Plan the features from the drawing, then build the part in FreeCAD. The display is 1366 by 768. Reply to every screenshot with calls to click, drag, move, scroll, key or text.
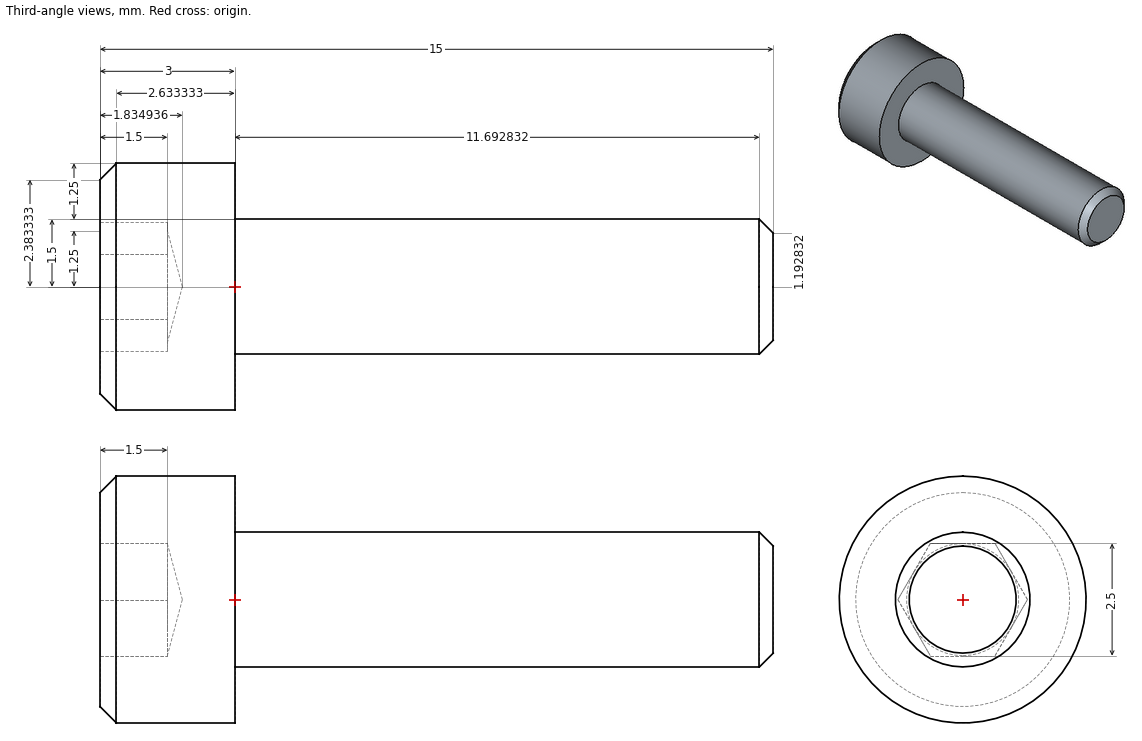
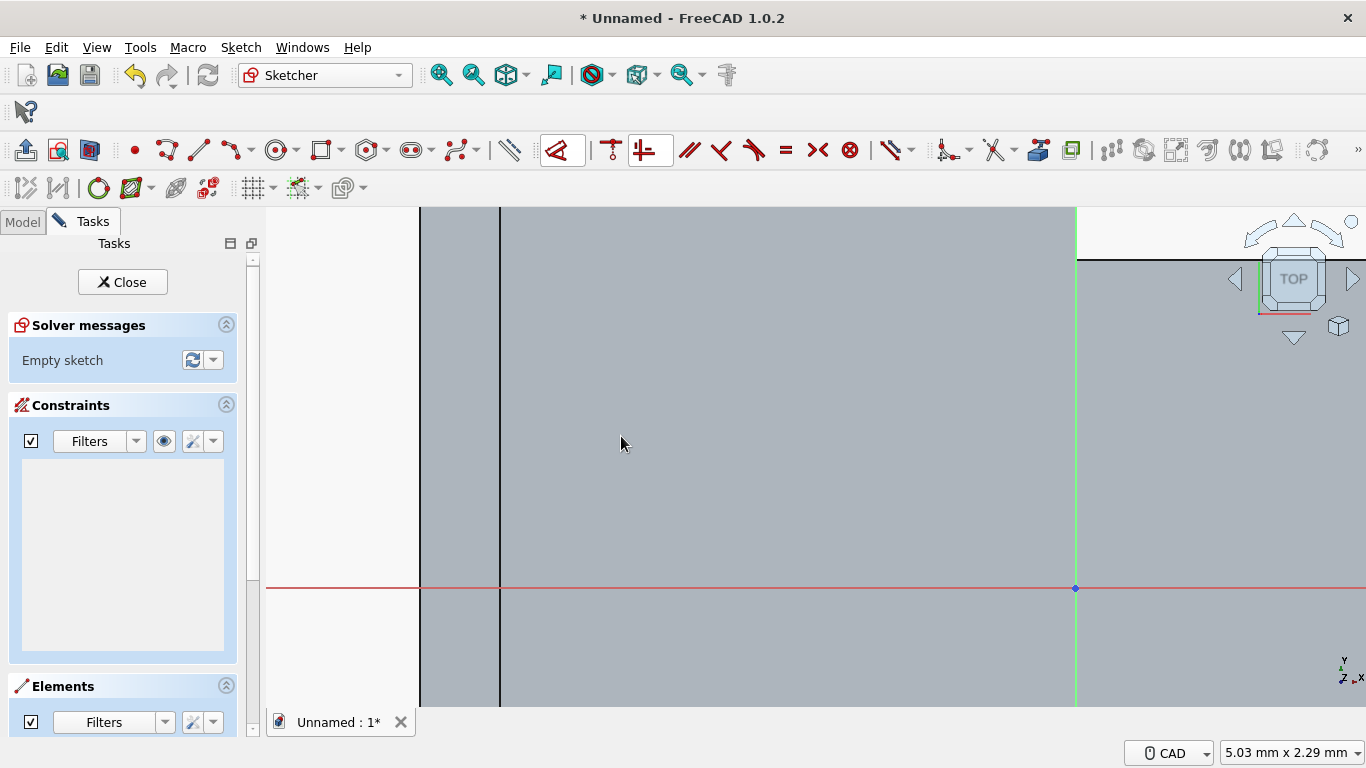
click(168, 150)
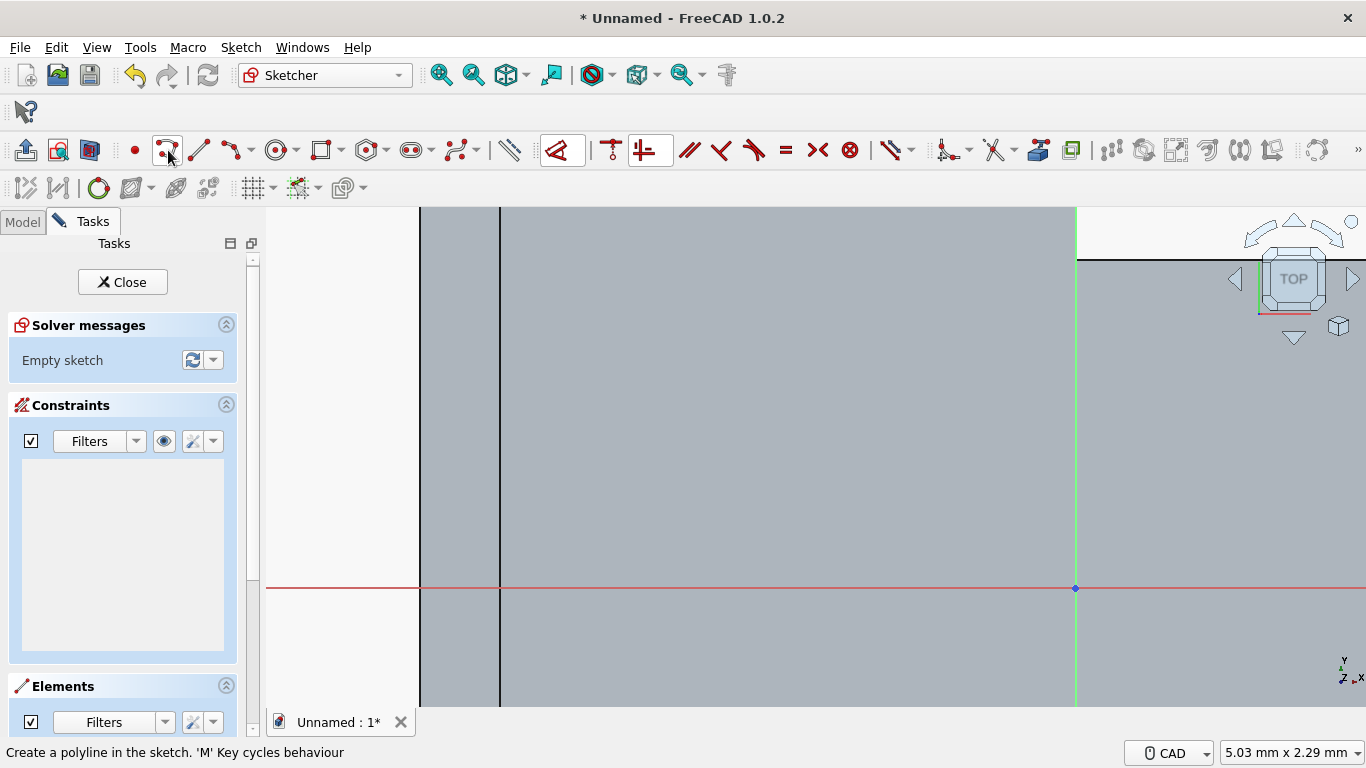
click(821, 588)
click(748, 315)
click(420, 315)
click(420, 579)
click(821, 588)
key(Escape)
key(Escape)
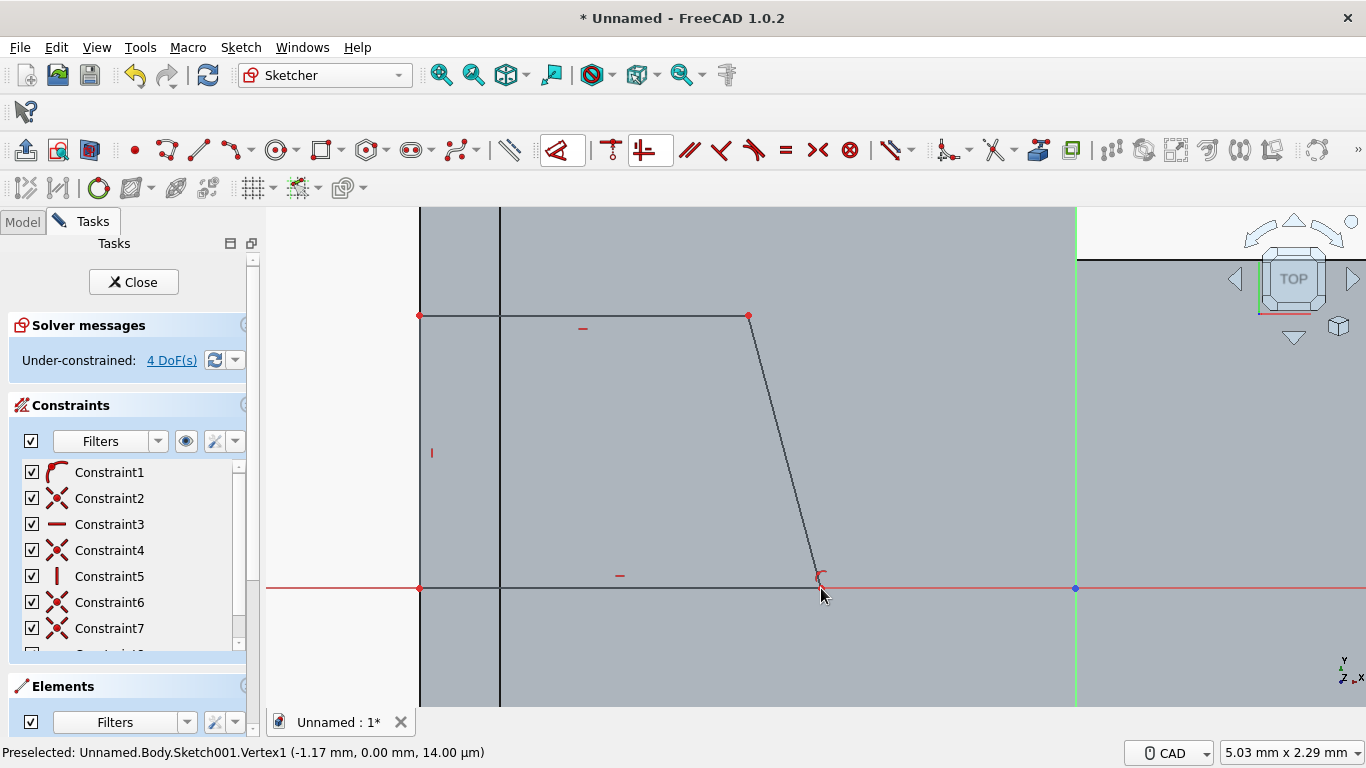
click(420, 316)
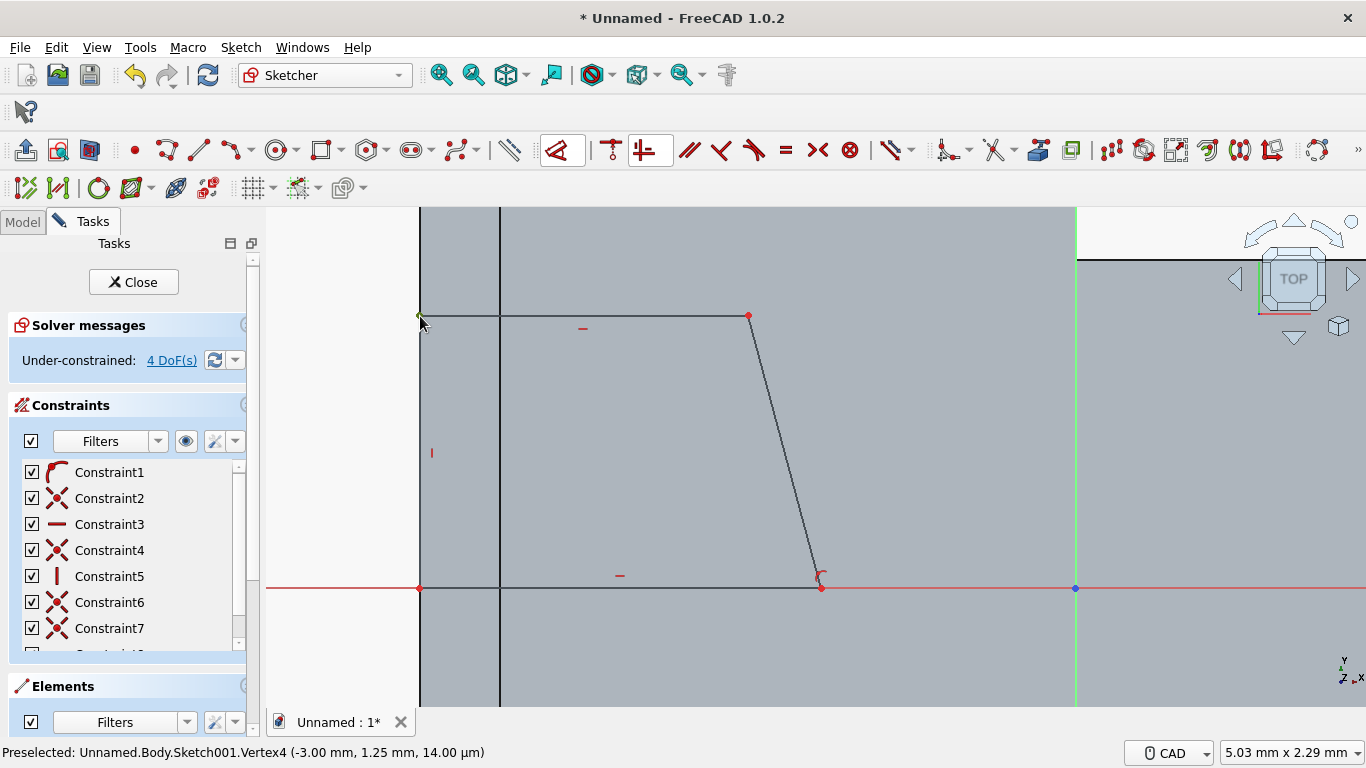
key(l)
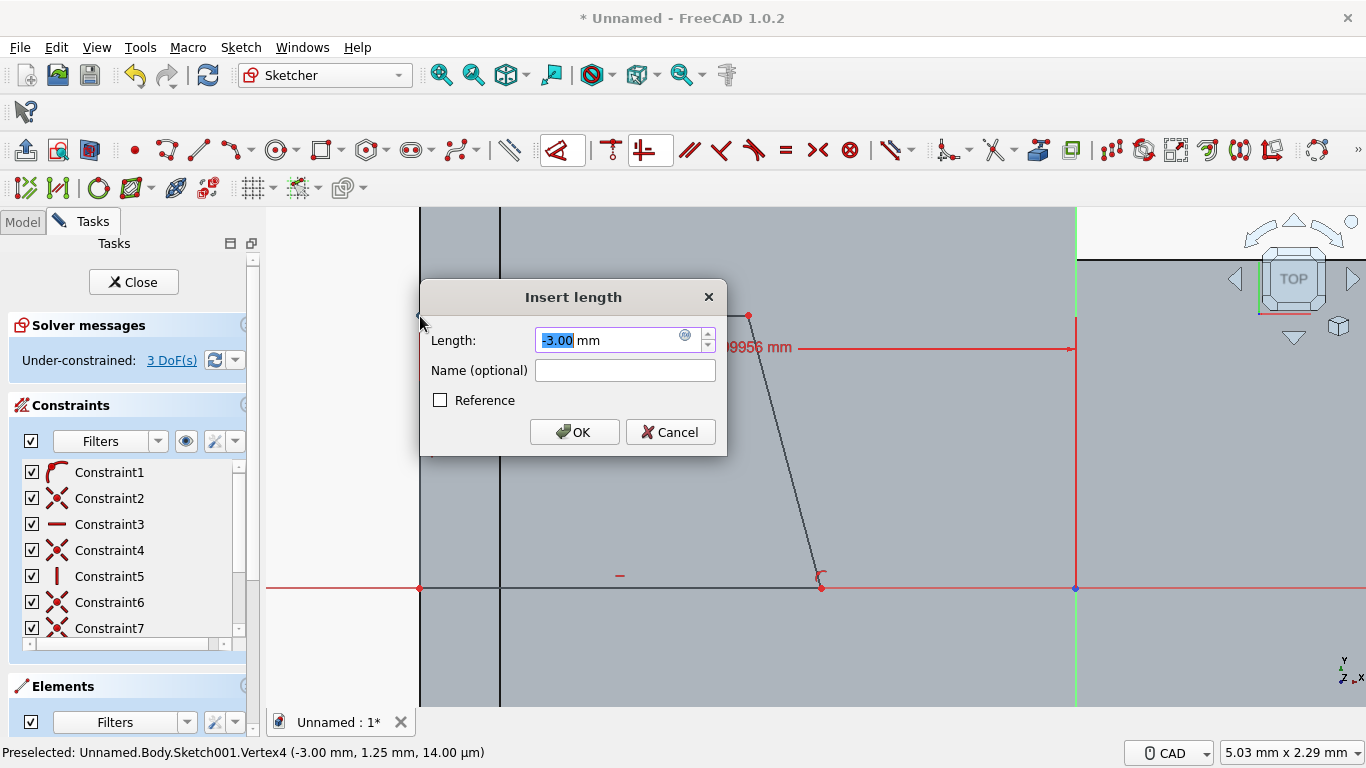
text(-3)
key(Return)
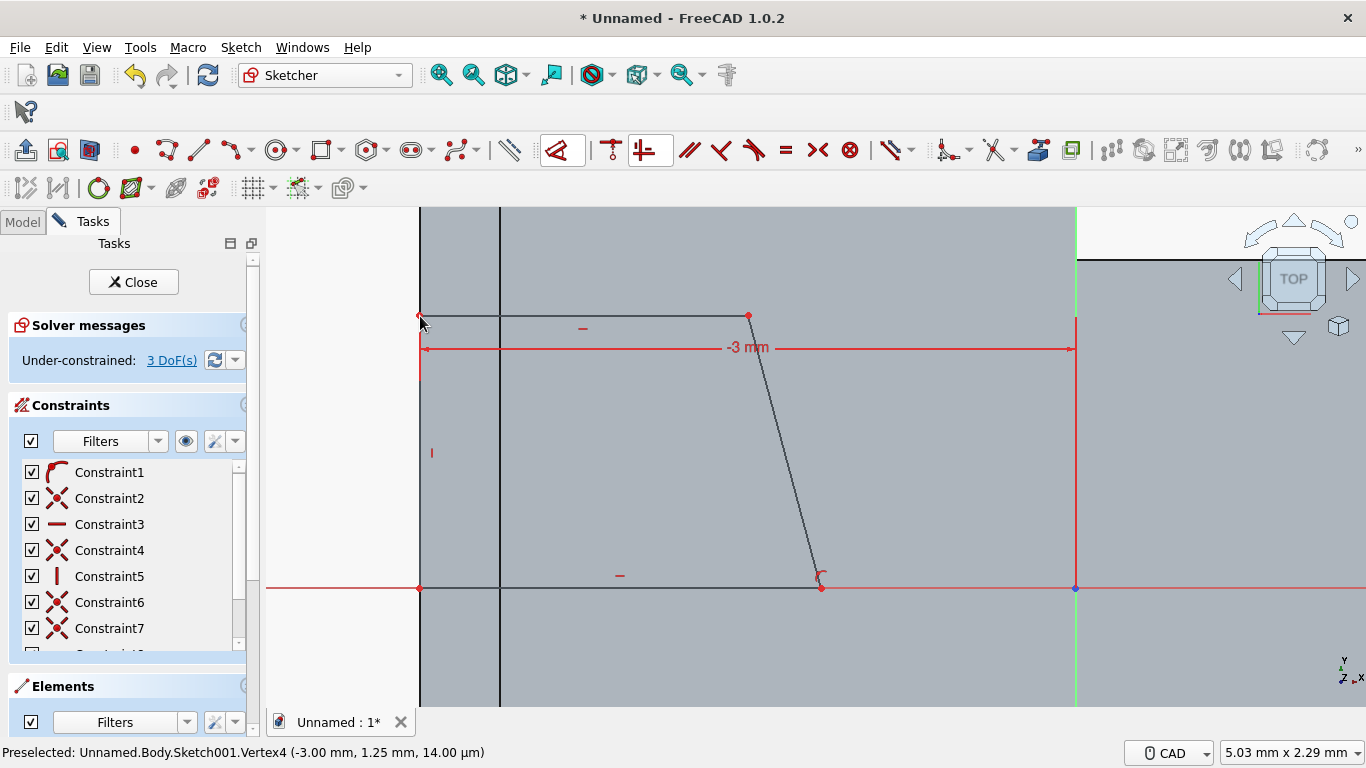
click(650, 316)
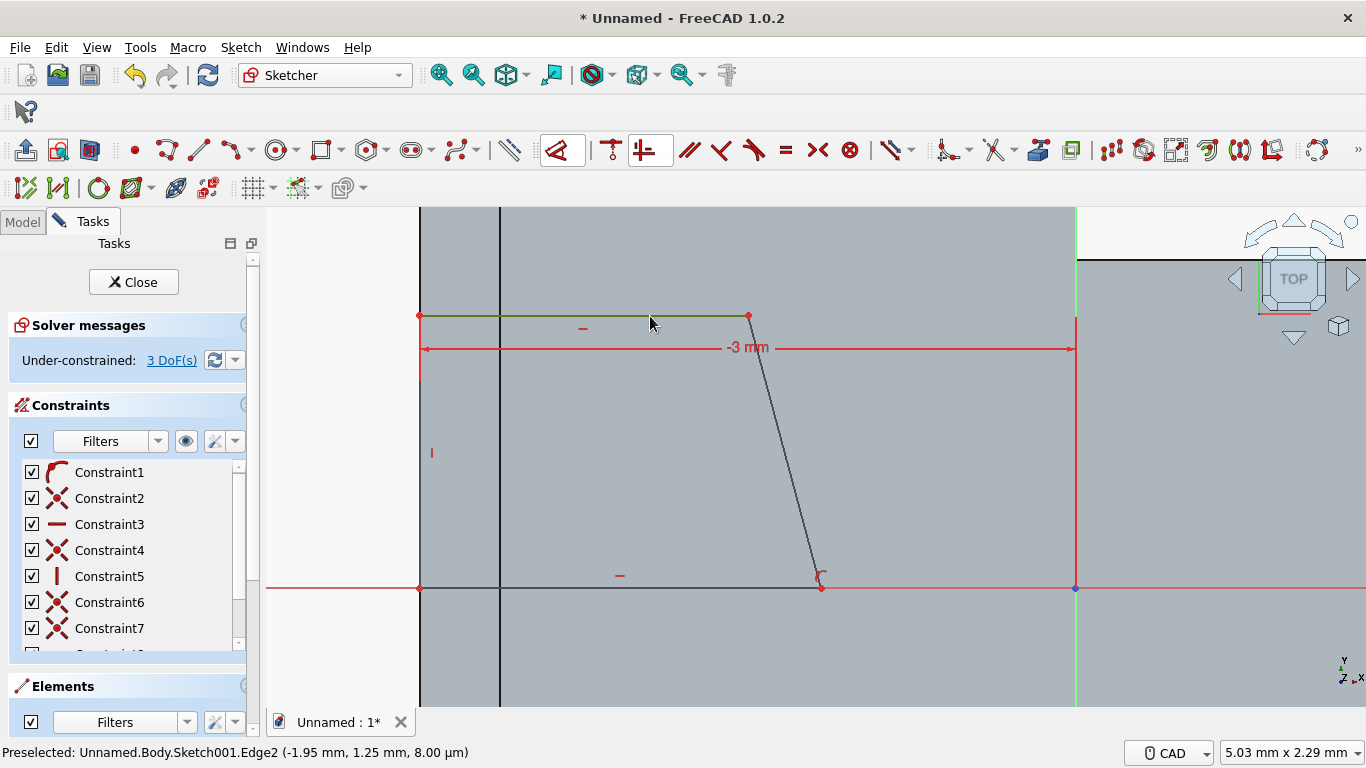
click(580, 150)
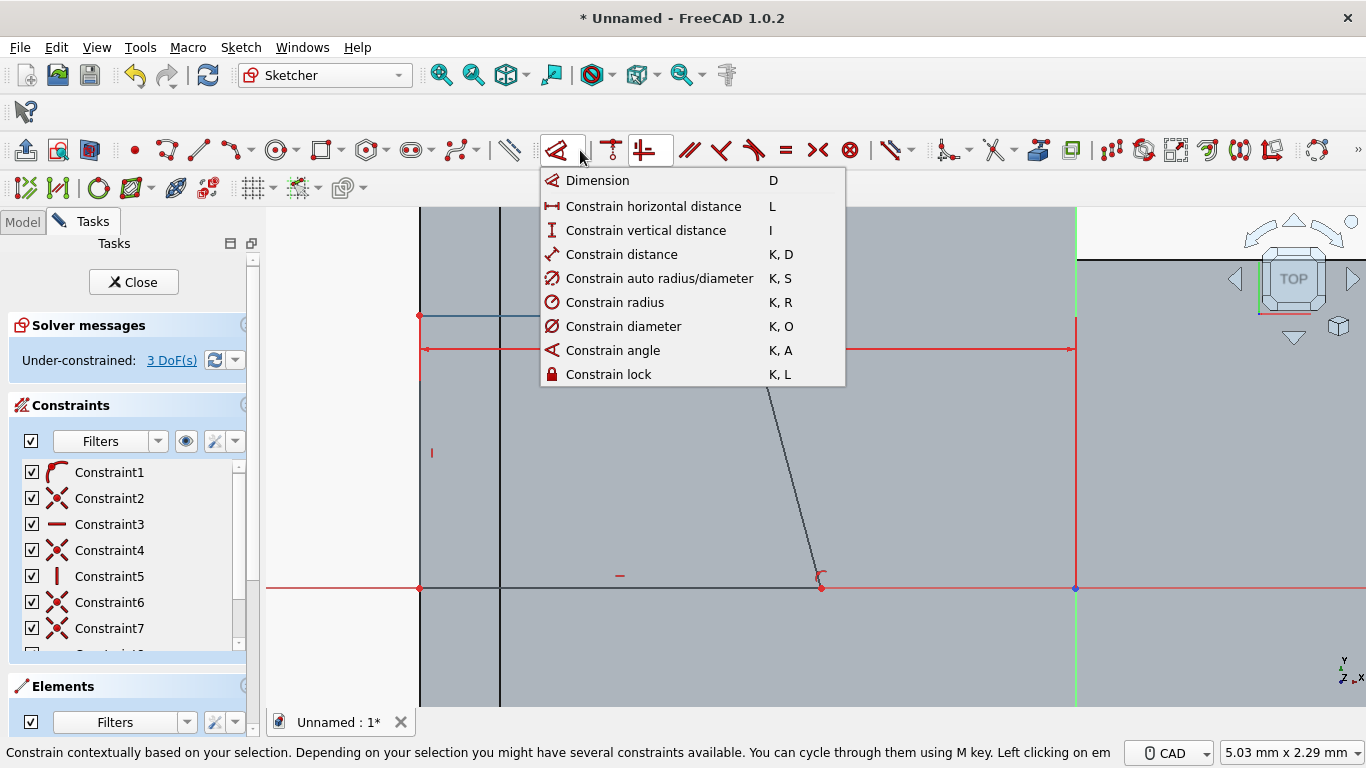
click(693, 206)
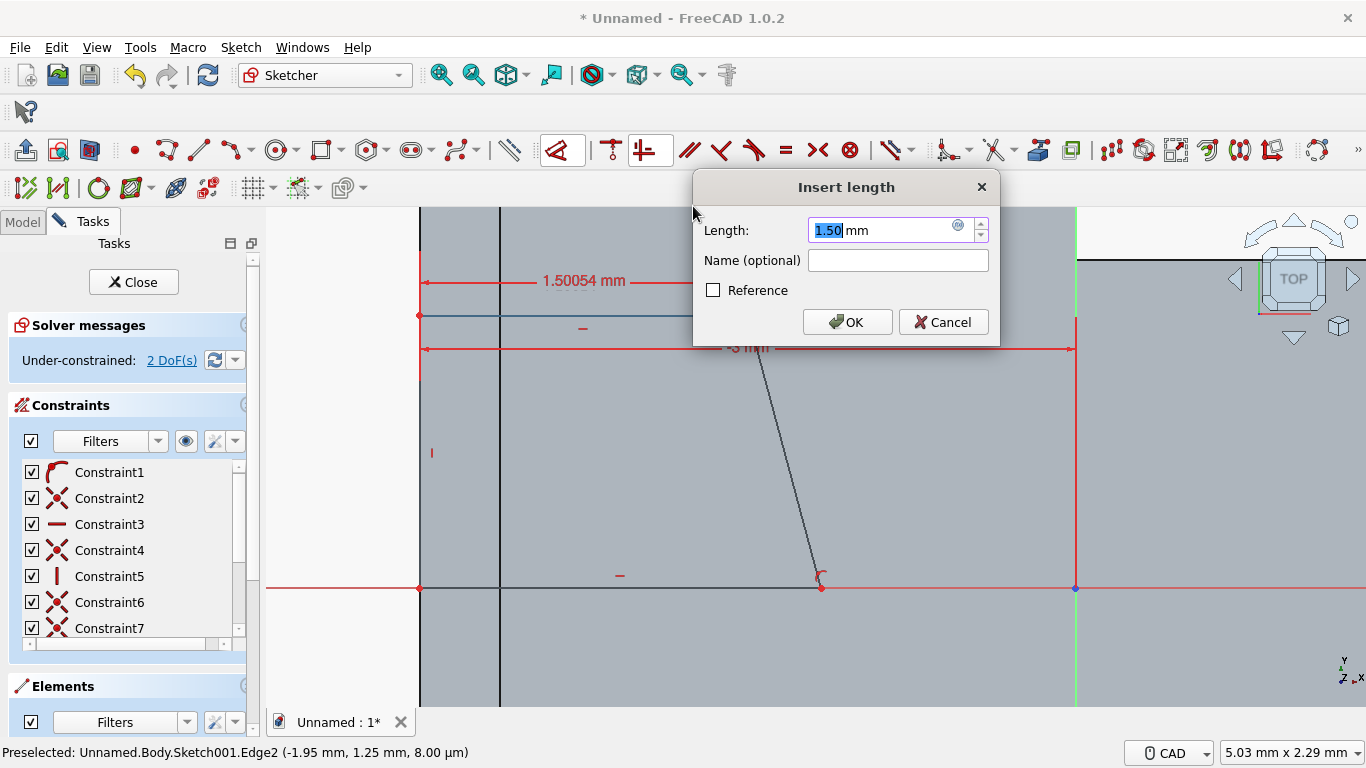
text(1.5)
key(Return)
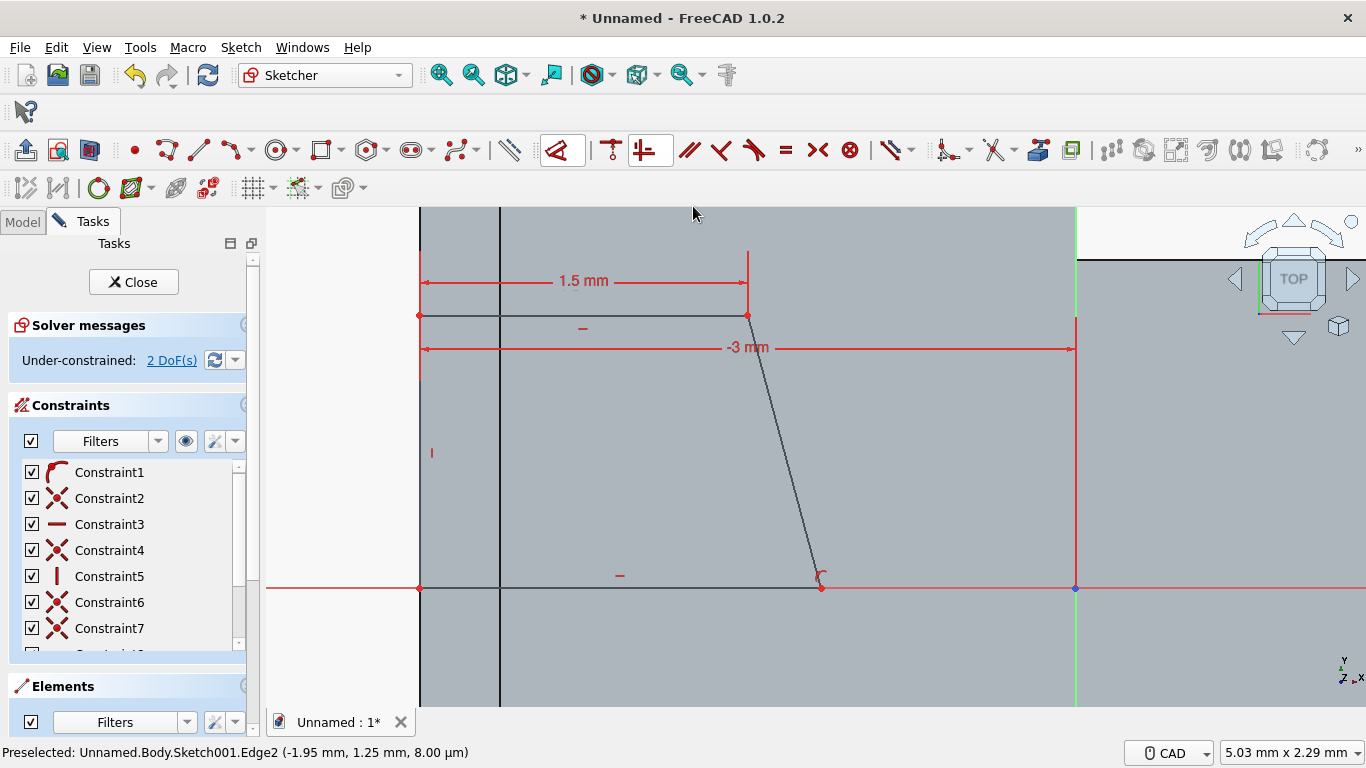
click(420, 398)